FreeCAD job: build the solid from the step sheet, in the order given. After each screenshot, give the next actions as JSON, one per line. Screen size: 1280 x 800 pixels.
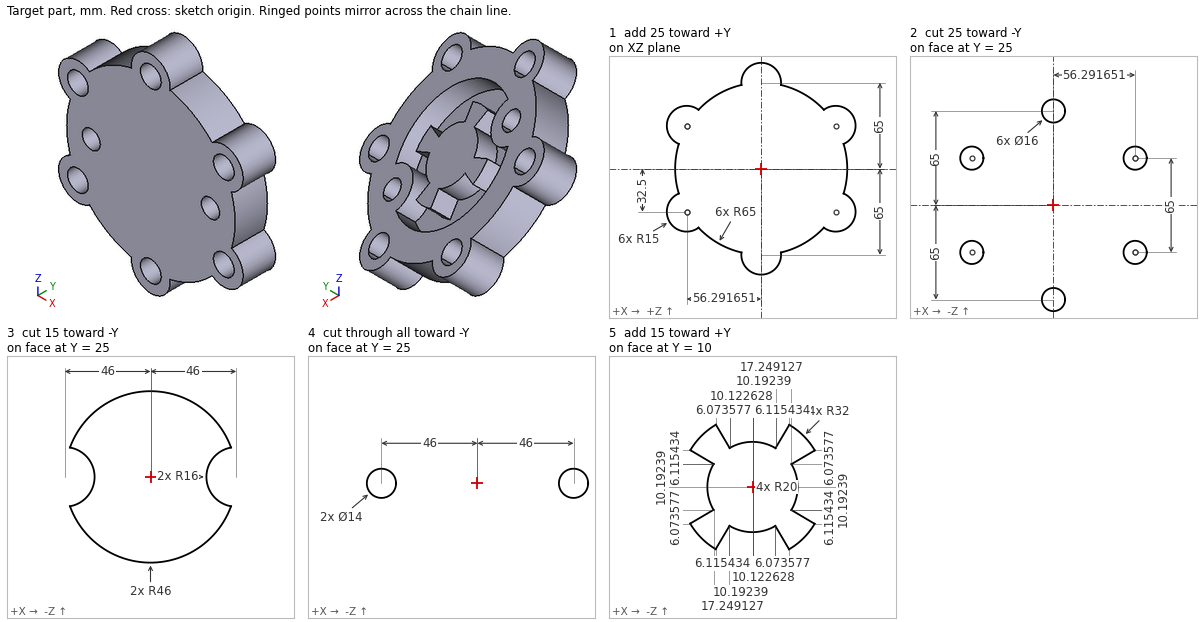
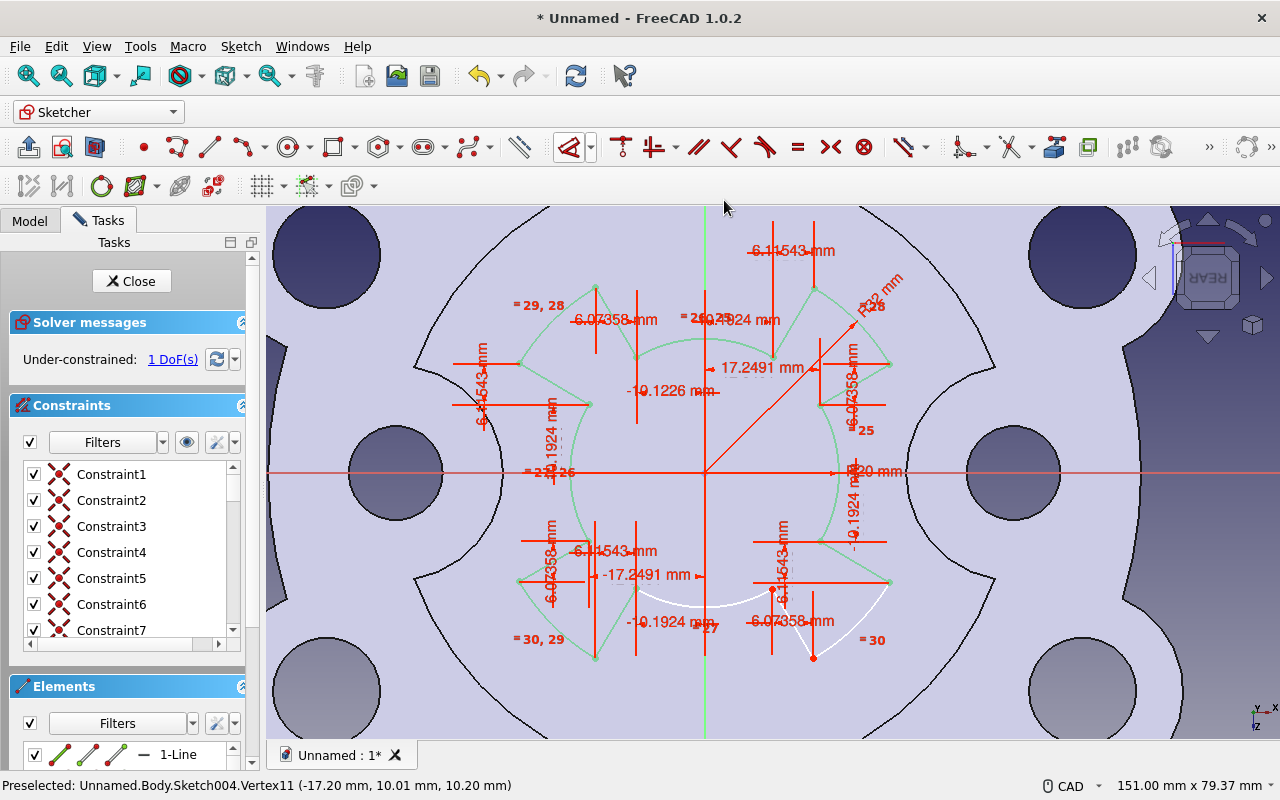
{"action": "left_click", "coordinate": [772, 589]}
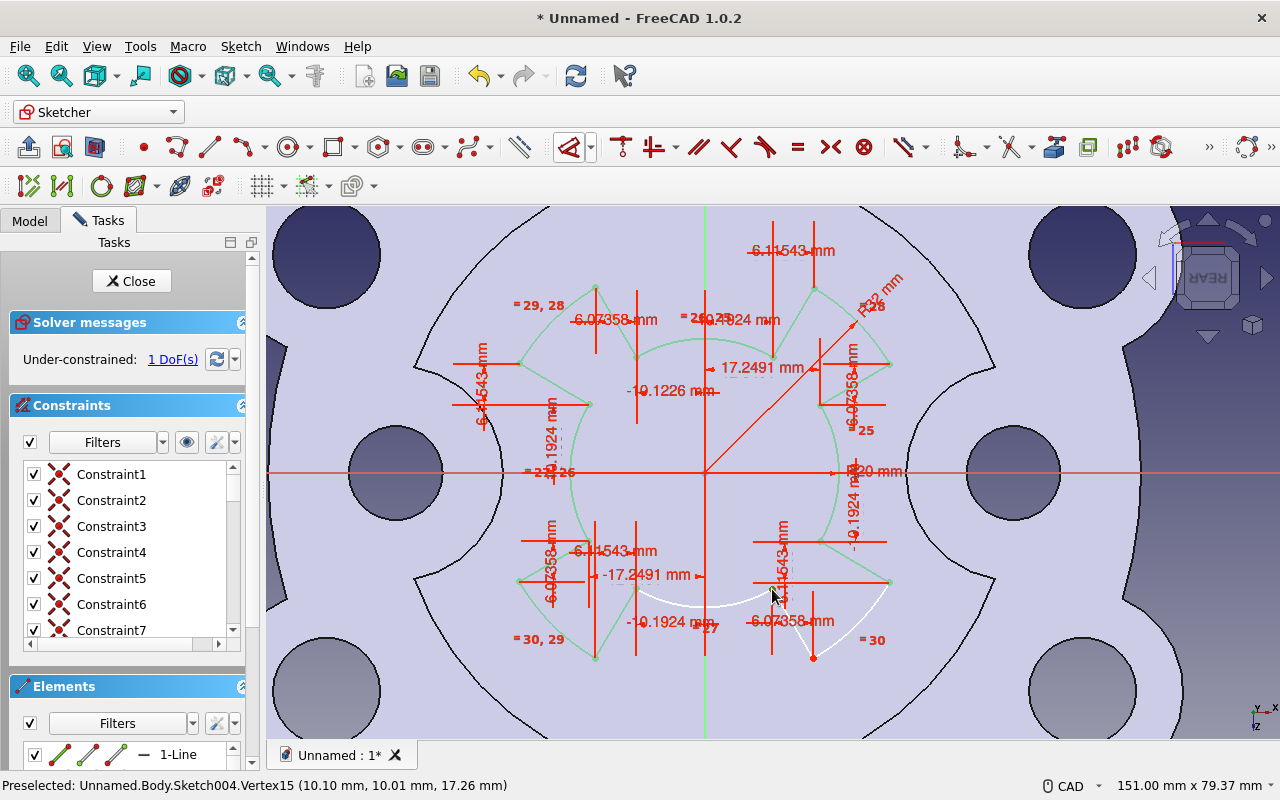
{"action": "key", "text": "l"}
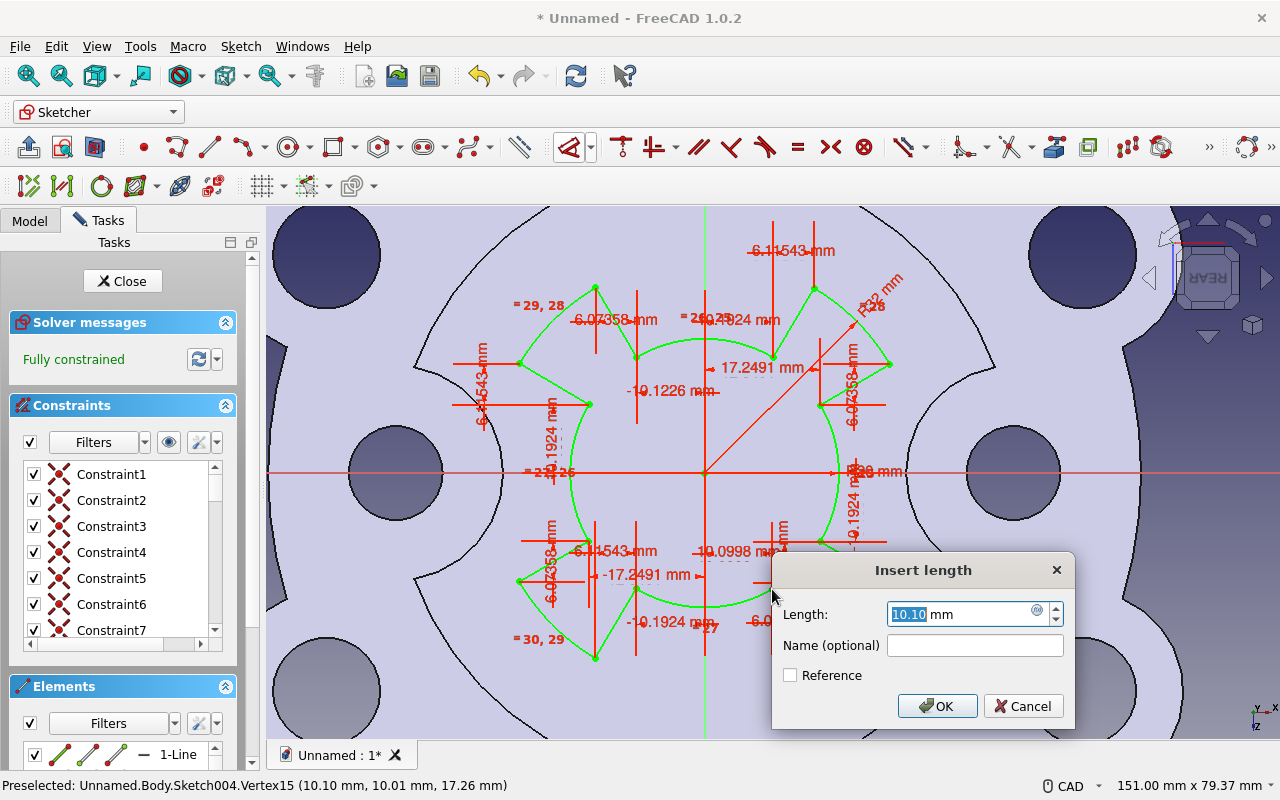
{"action": "type", "text": "10.122628"}
{"action": "key", "text": "Return"}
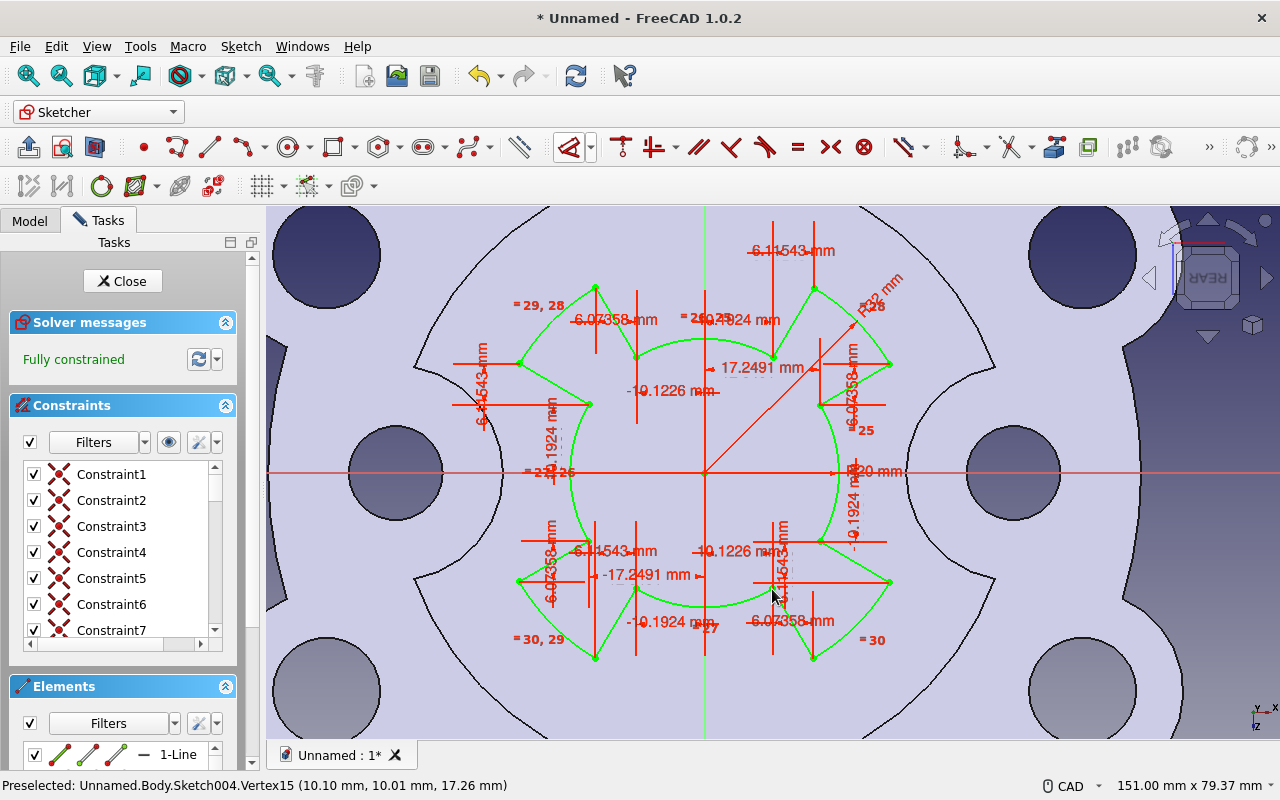
{"action": "left_click", "coordinate": [123, 281]}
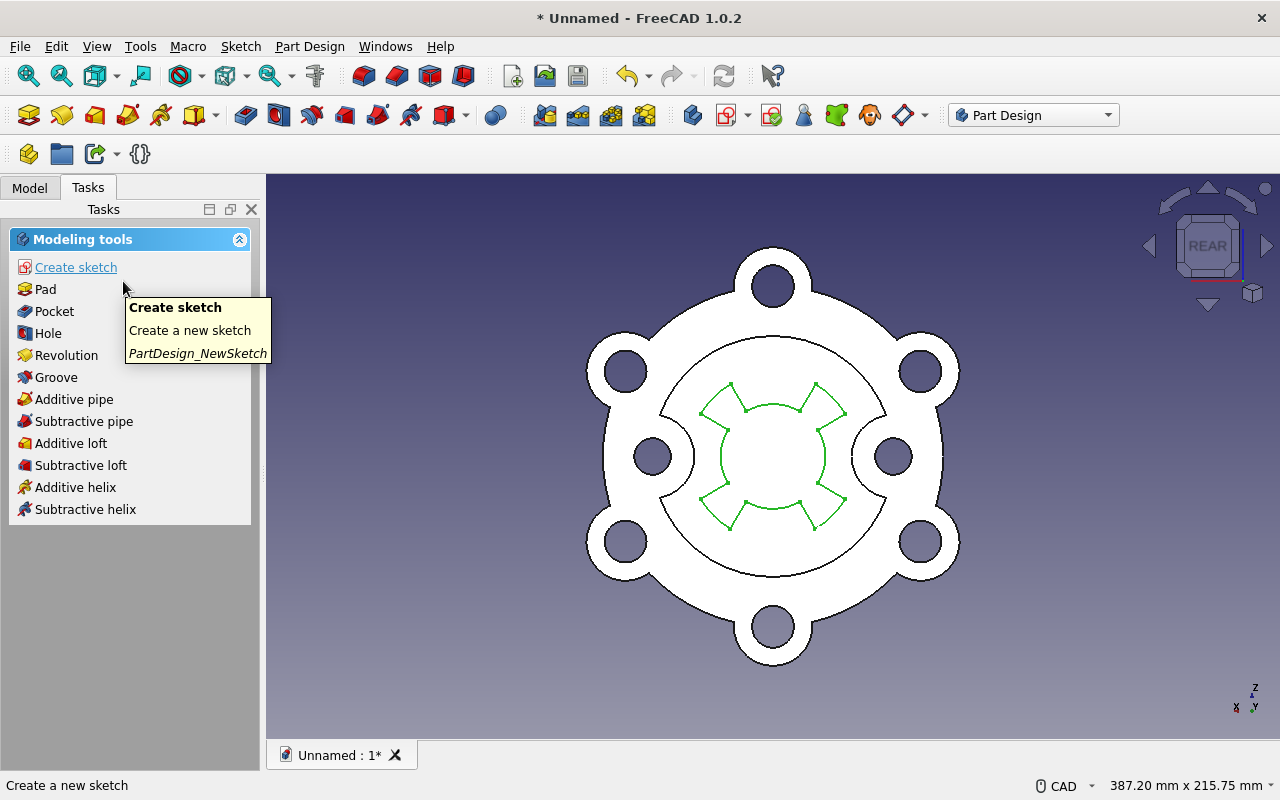
{"action": "left_click", "coordinate": [29, 116]}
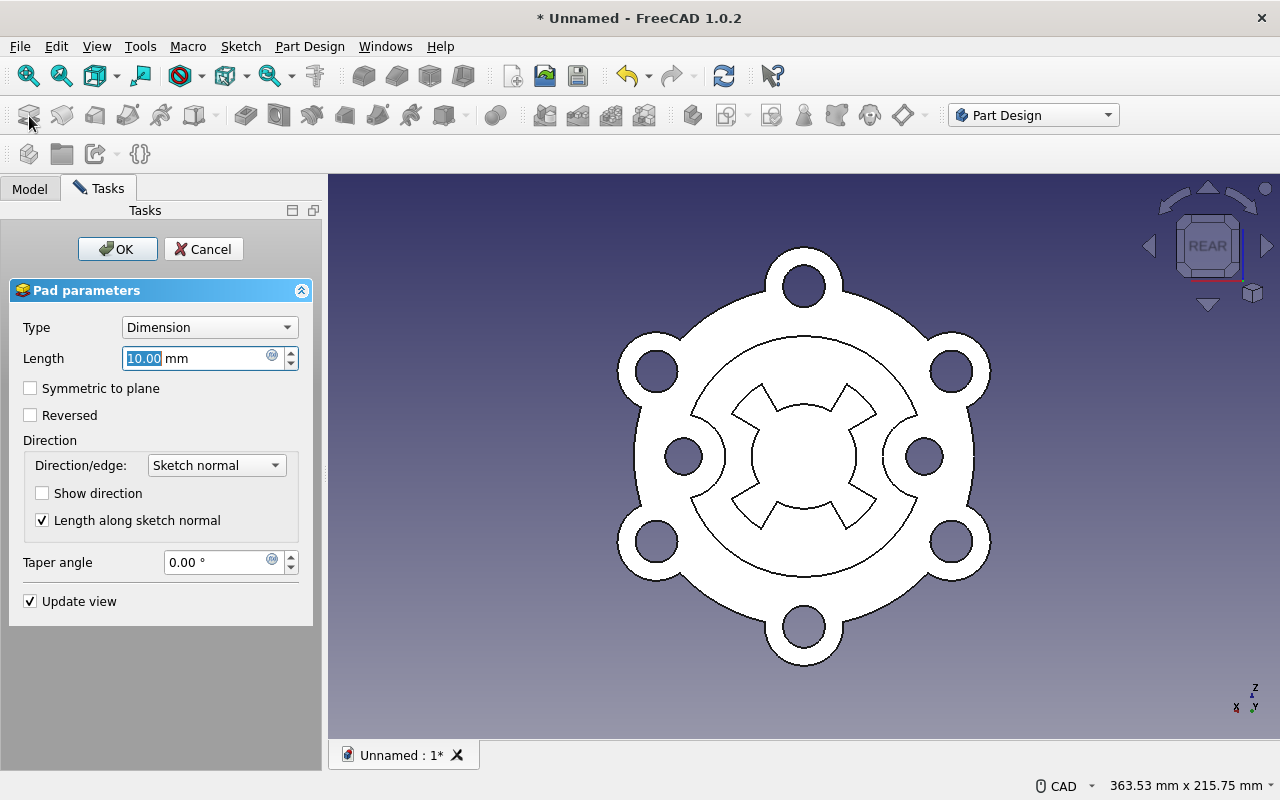
{"action": "type", "text": "15"}
{"action": "key", "text": "Tab"}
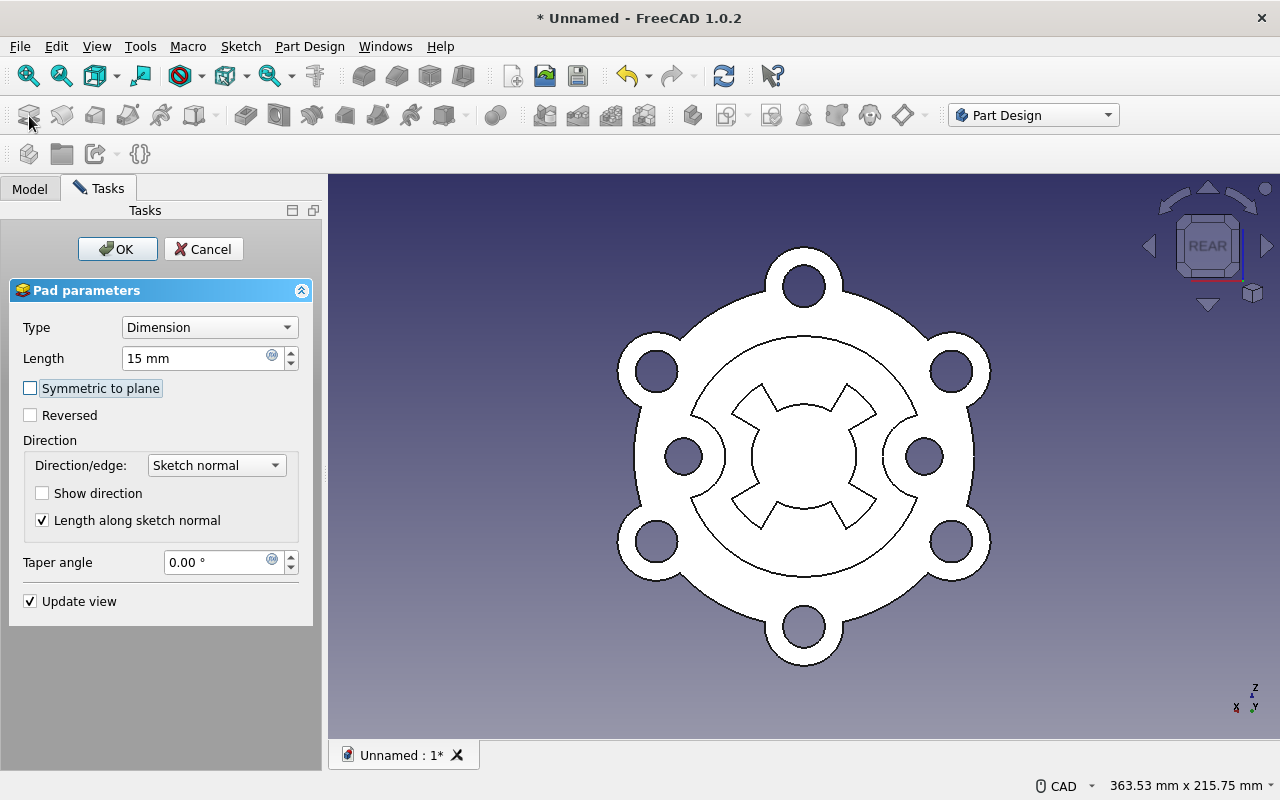
{"action": "left_click", "coordinate": [118, 249]}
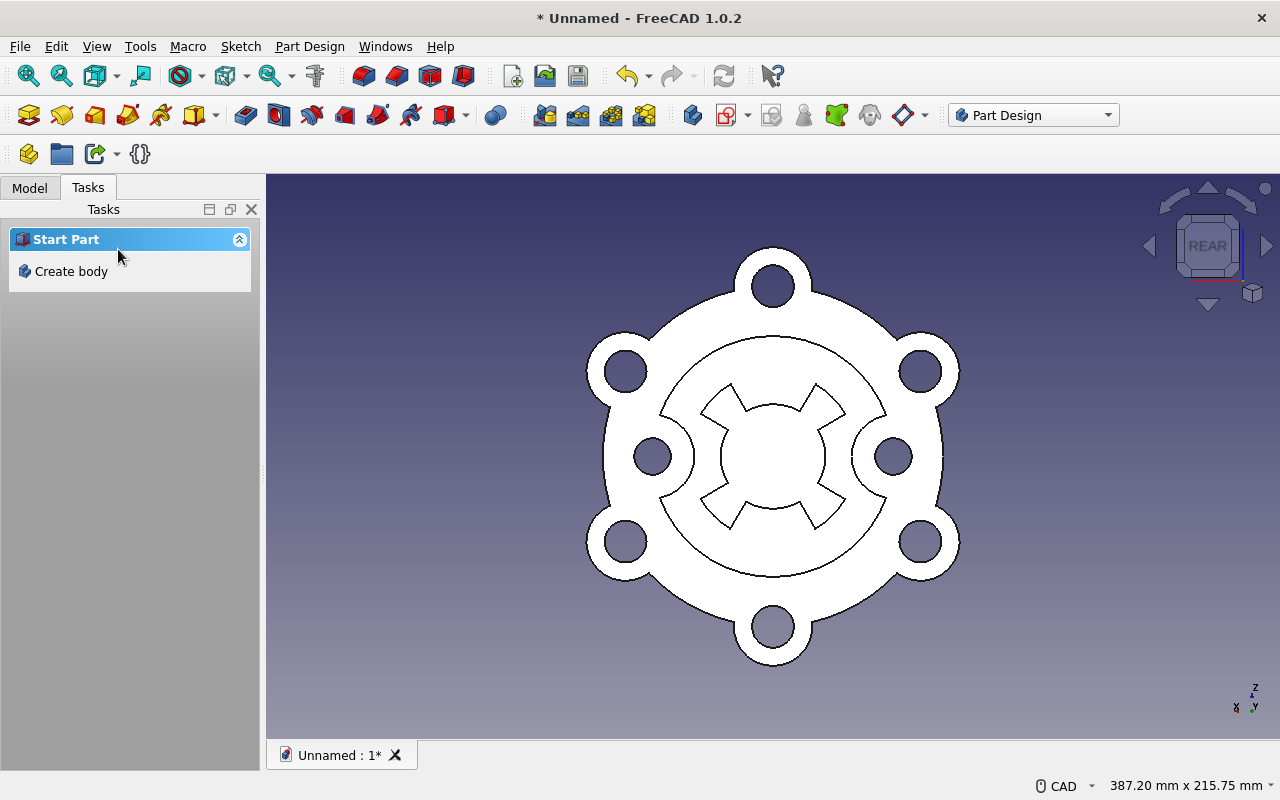
{"action": "key", "text": "0"}